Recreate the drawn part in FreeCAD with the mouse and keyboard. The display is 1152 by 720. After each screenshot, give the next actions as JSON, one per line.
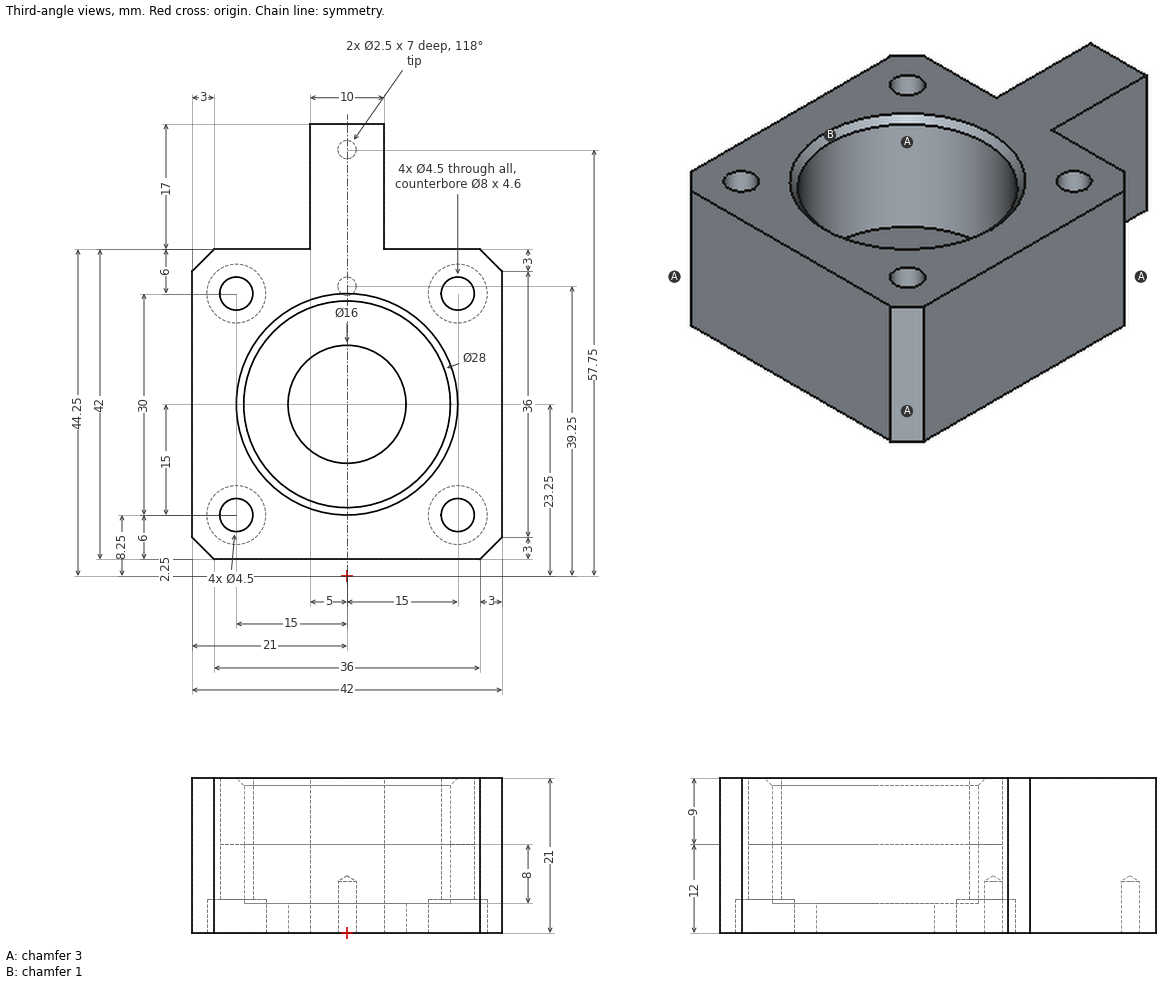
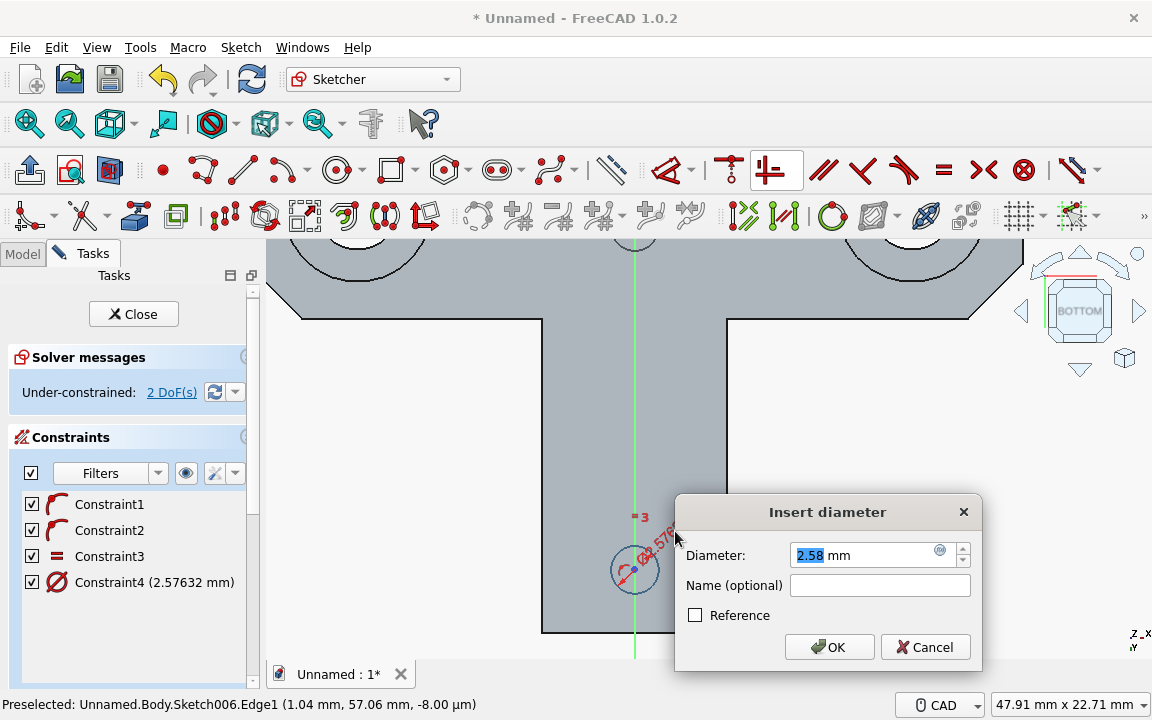
{"action": "type", "text": "2.5"}
{"action": "key", "text": "Return"}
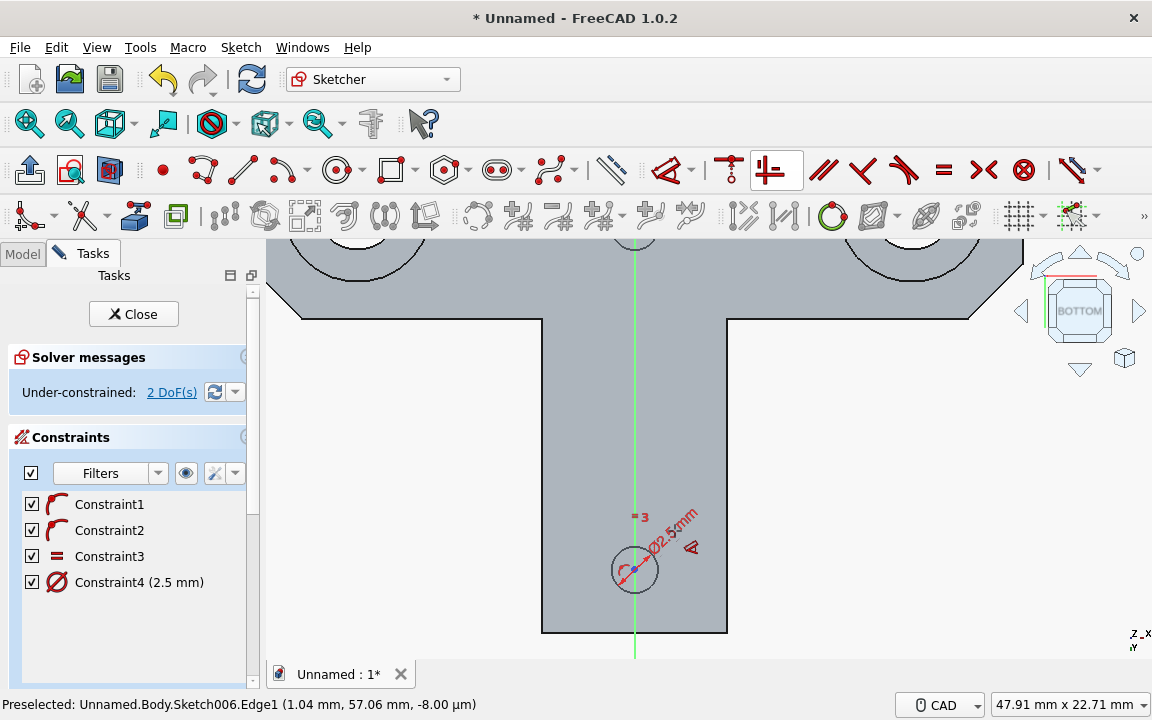
{"action": "left_click", "coordinate": [635, 570]}
{"action": "left_click", "coordinate": [669, 418]}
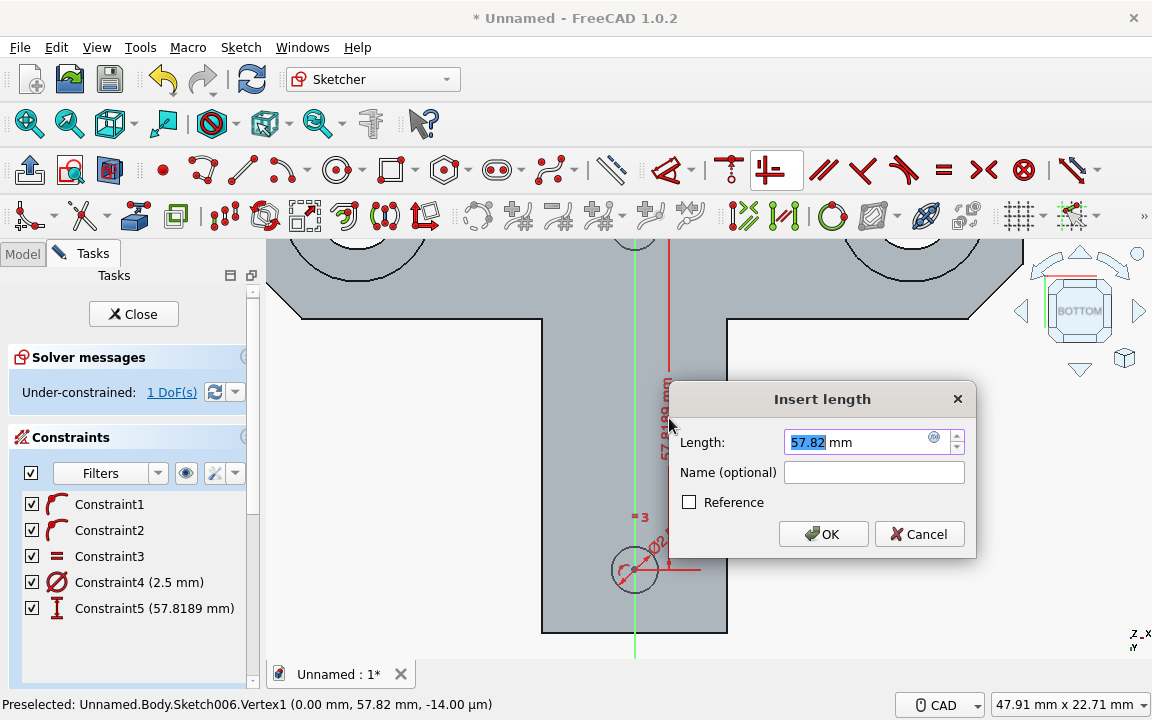
{"action": "type", "text": "57.75"}
{"action": "key", "text": "Return"}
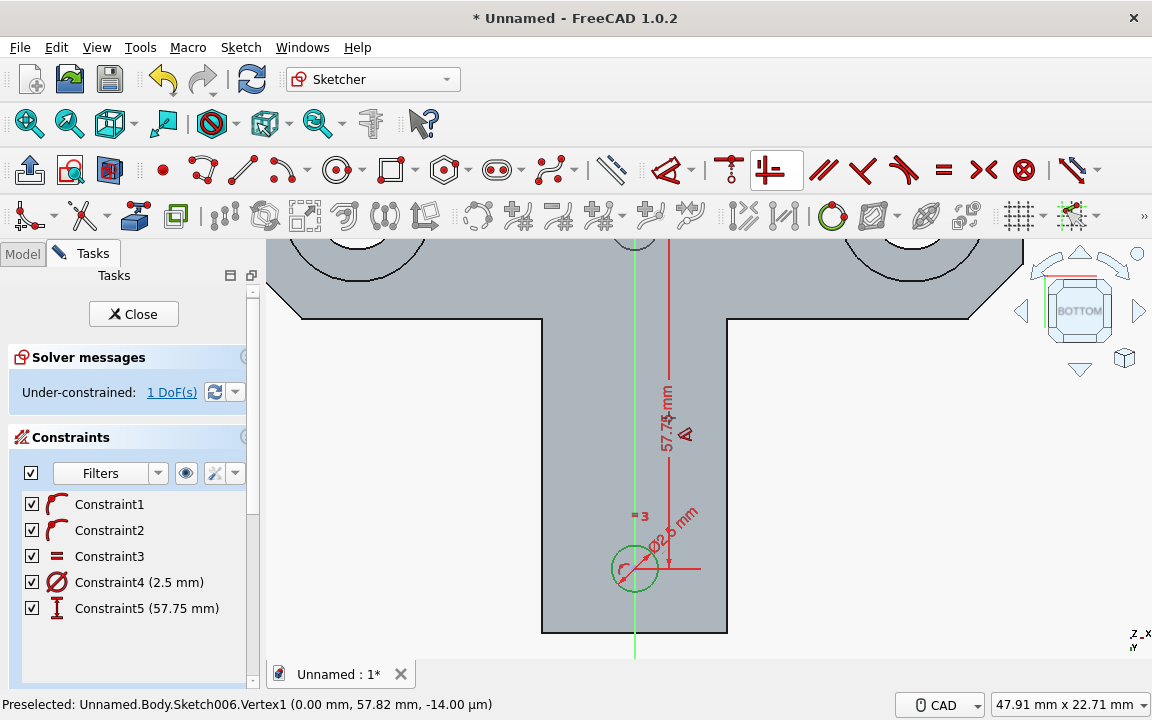
{"action": "scroll", "coordinate": [652, 554], "scroll_direction": "down", "scroll_amount": 2}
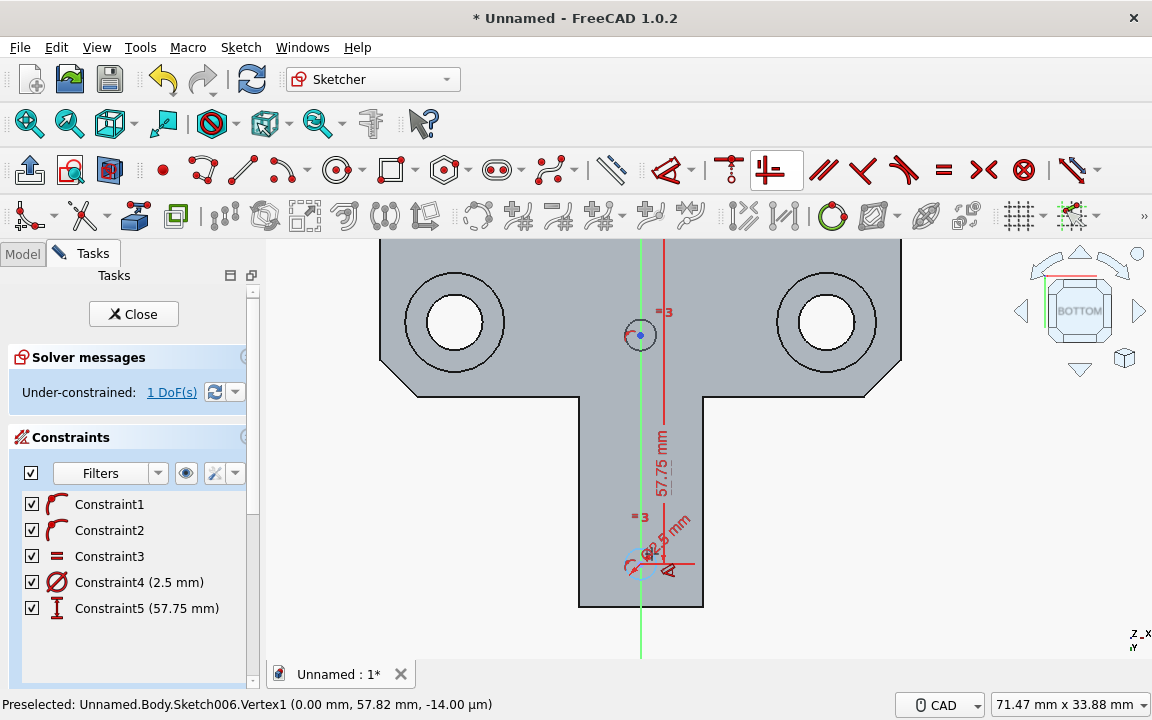
{"action": "left_click", "coordinate": [641, 335]}
{"action": "left_click", "coordinate": [675, 301]}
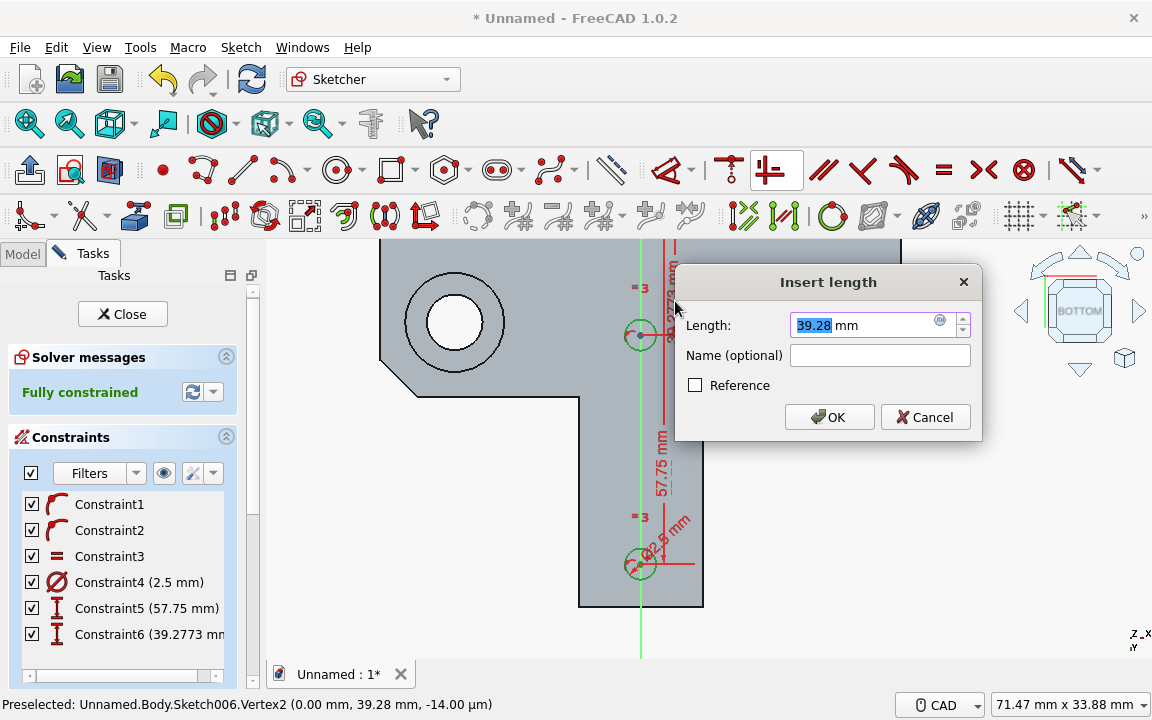
{"action": "type", "text": "39.25"}
{"action": "key", "text": "Return"}
{"action": "key", "text": "Escape"}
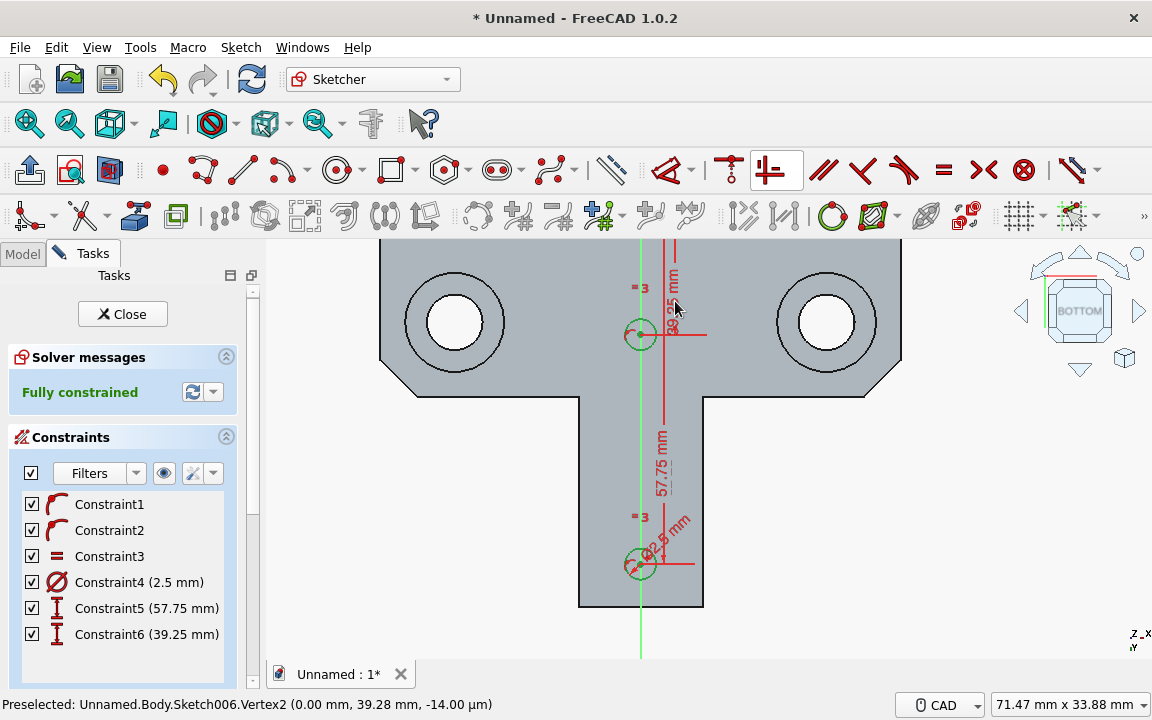
{"action": "left_click", "coordinate": [123, 314]}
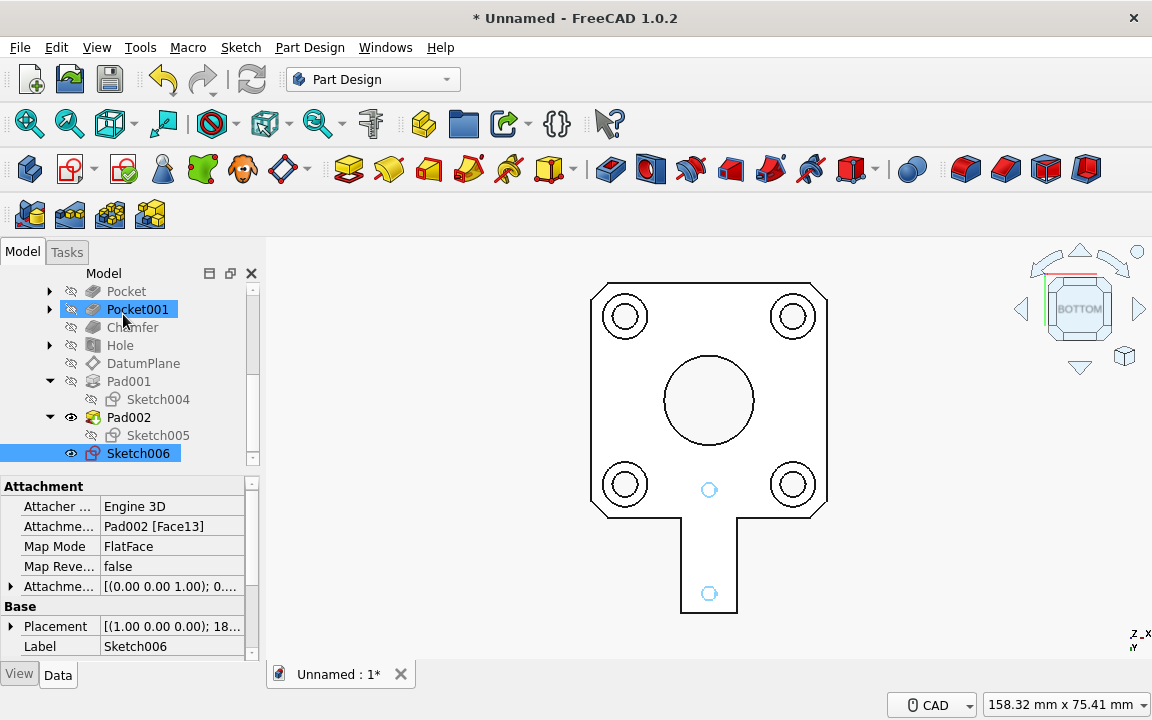
{"action": "left_click", "coordinate": [652, 170]}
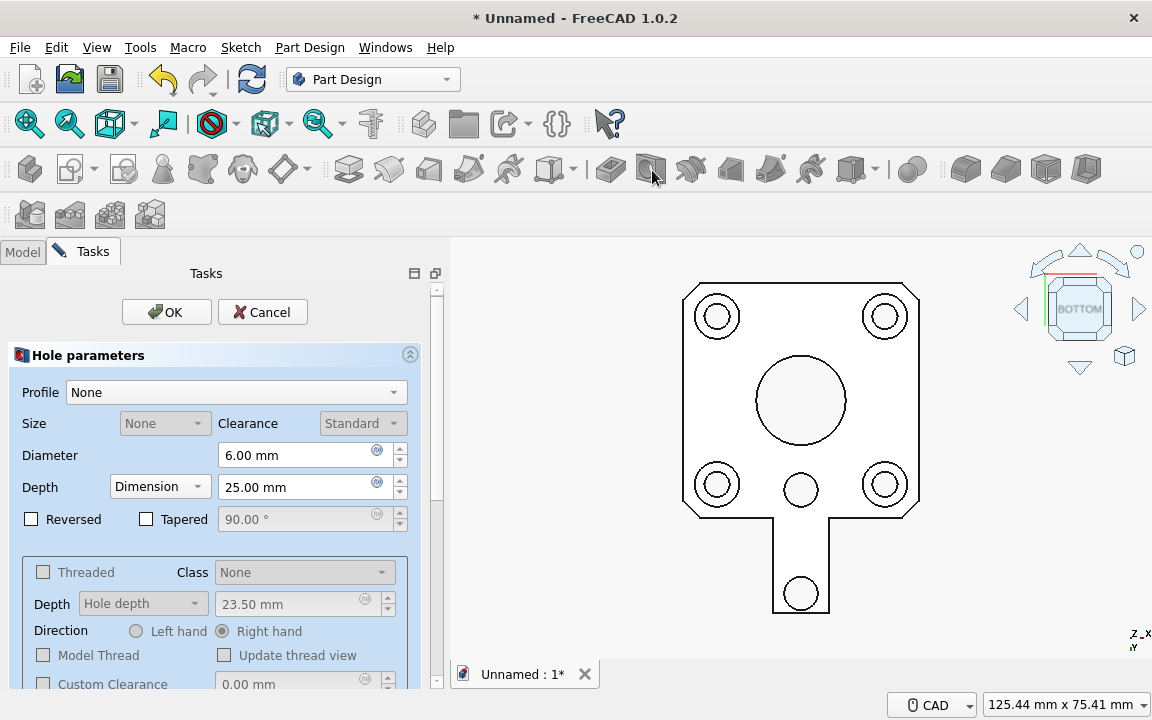
{"action": "triple_click", "coordinate": [305, 455]}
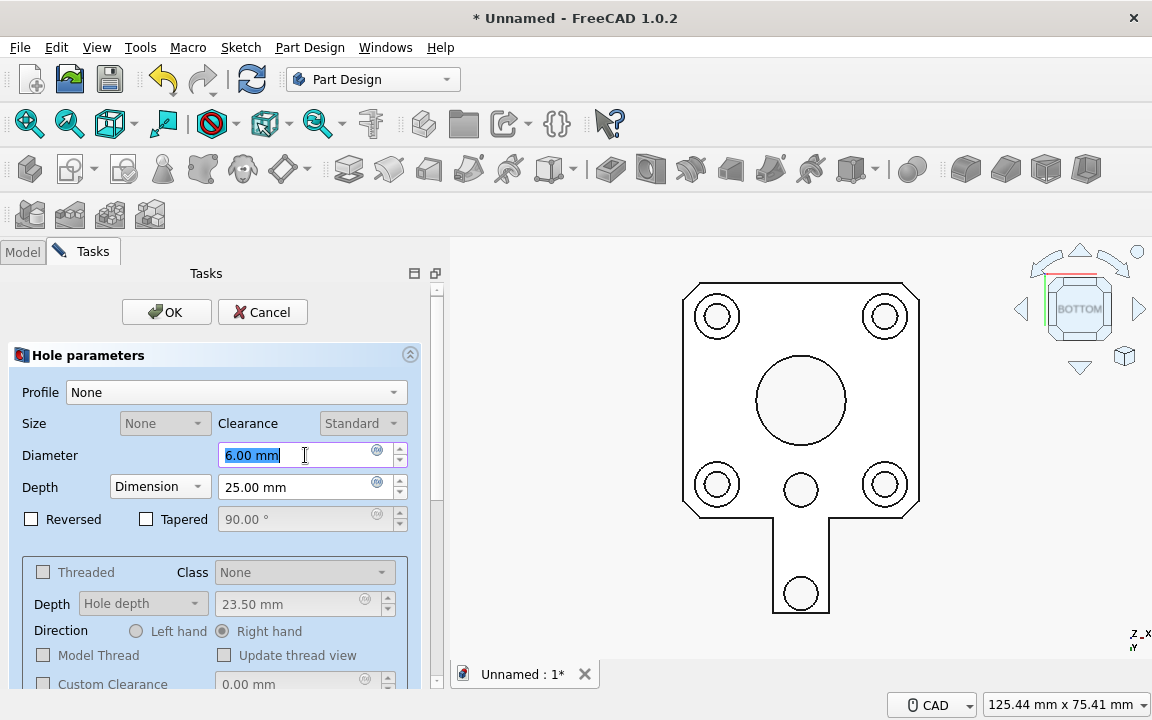
{"action": "type", "text": "2.5"}
{"action": "key", "text": "Tab"}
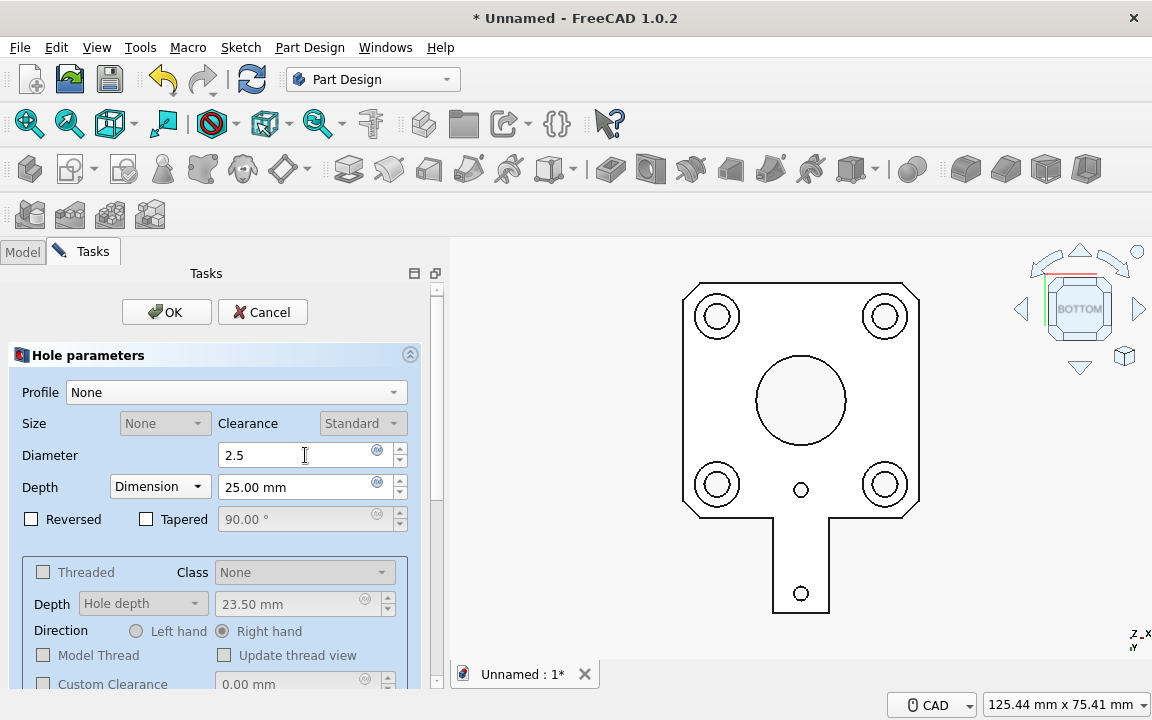
{"action": "triple_click", "coordinate": [305, 487]}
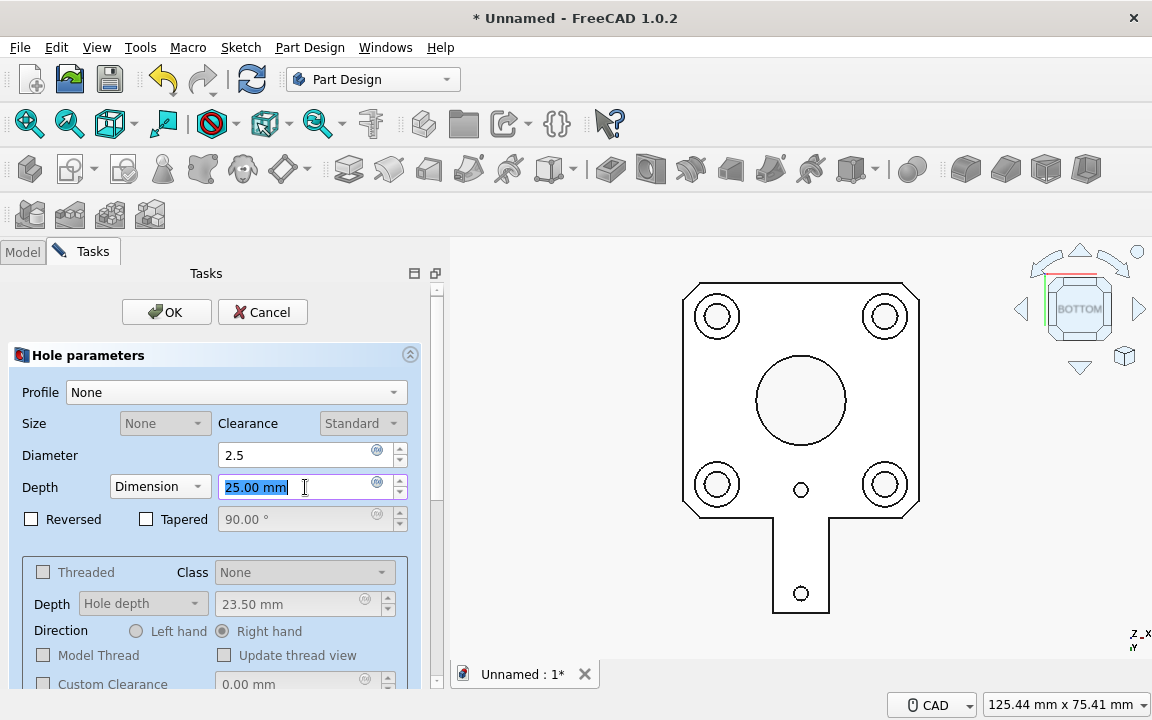
{"action": "type", "text": "7"}
{"action": "key", "text": "Tab"}